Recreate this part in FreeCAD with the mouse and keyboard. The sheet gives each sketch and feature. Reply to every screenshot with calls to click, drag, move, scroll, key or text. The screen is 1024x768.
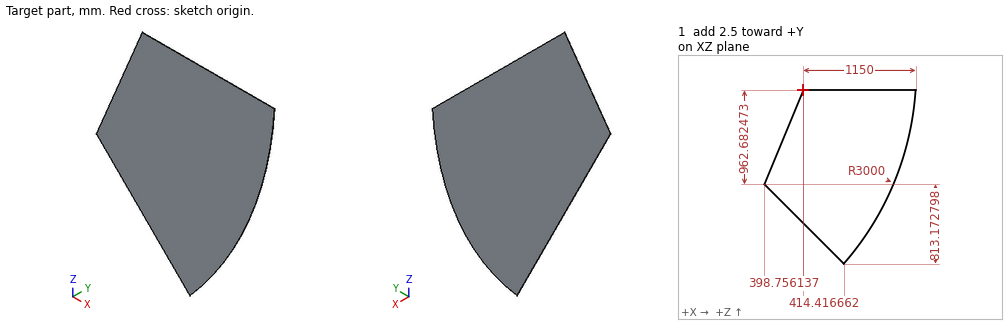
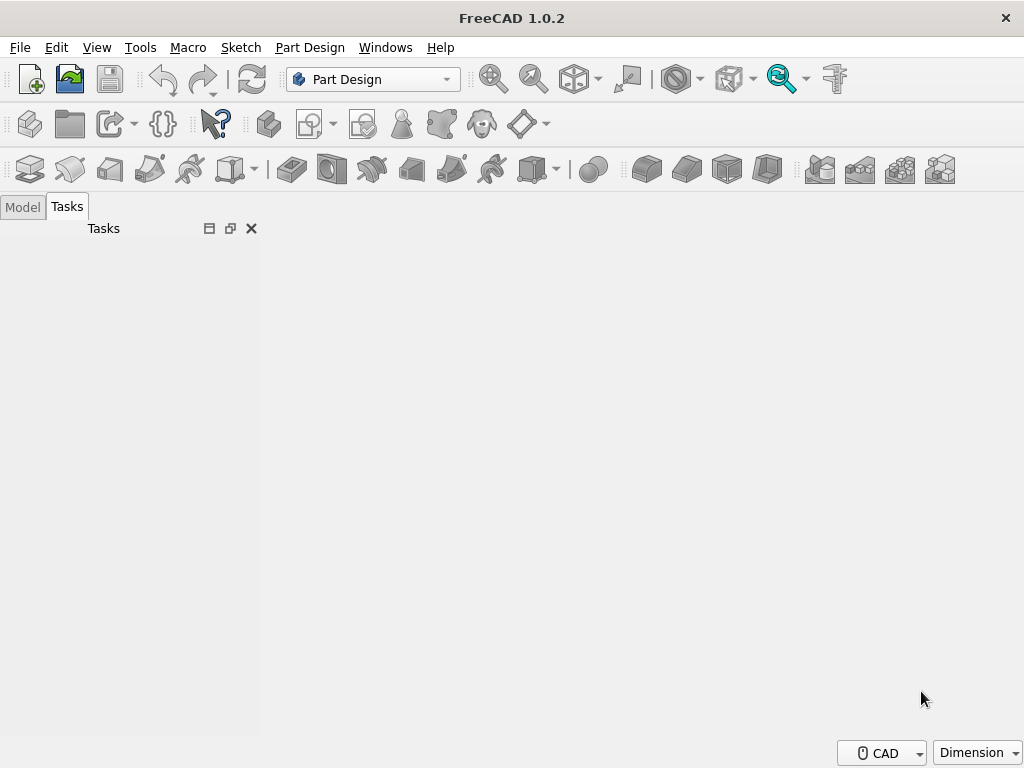
key(ctrl+n)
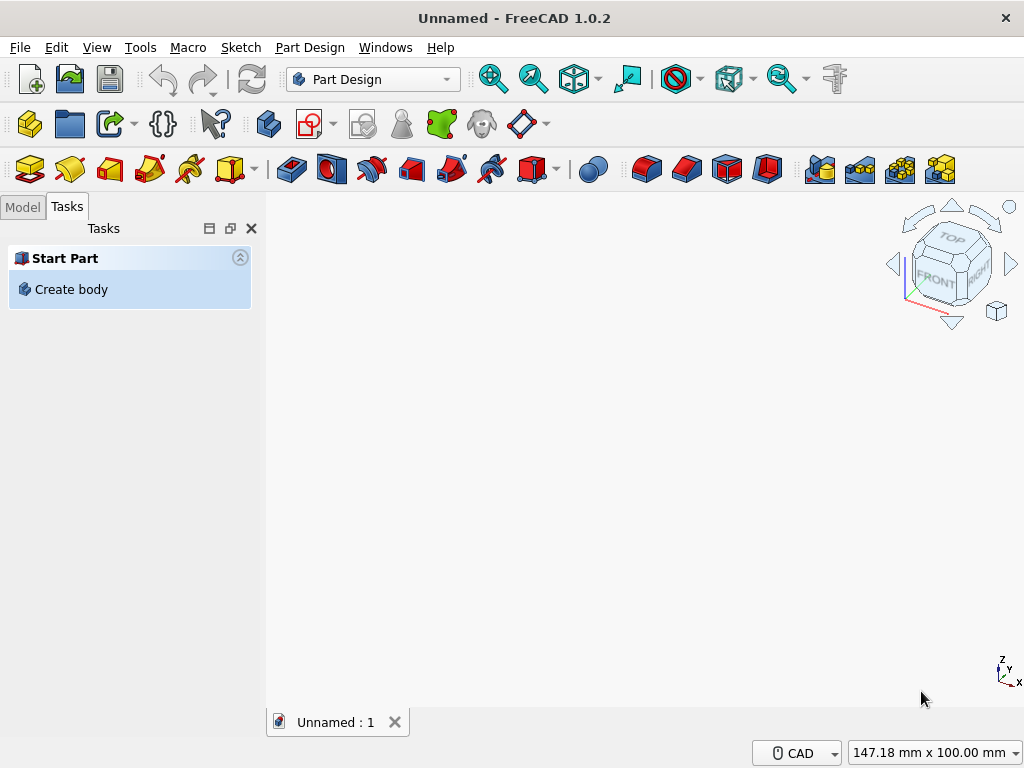
click(310, 124)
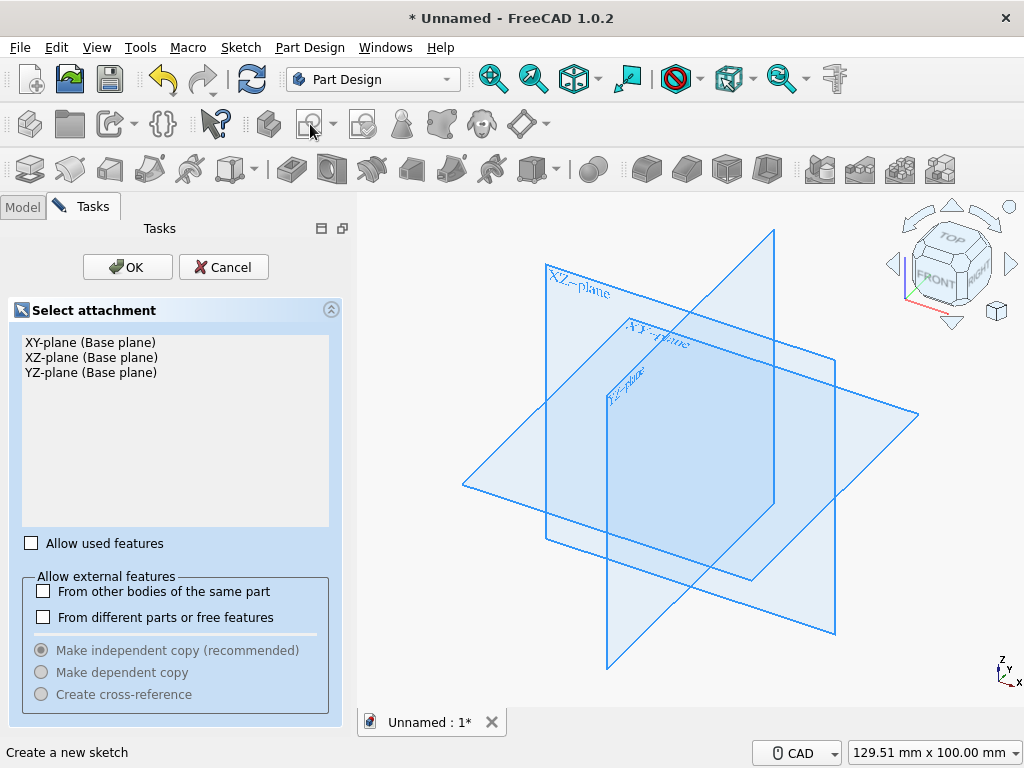
click(82, 358)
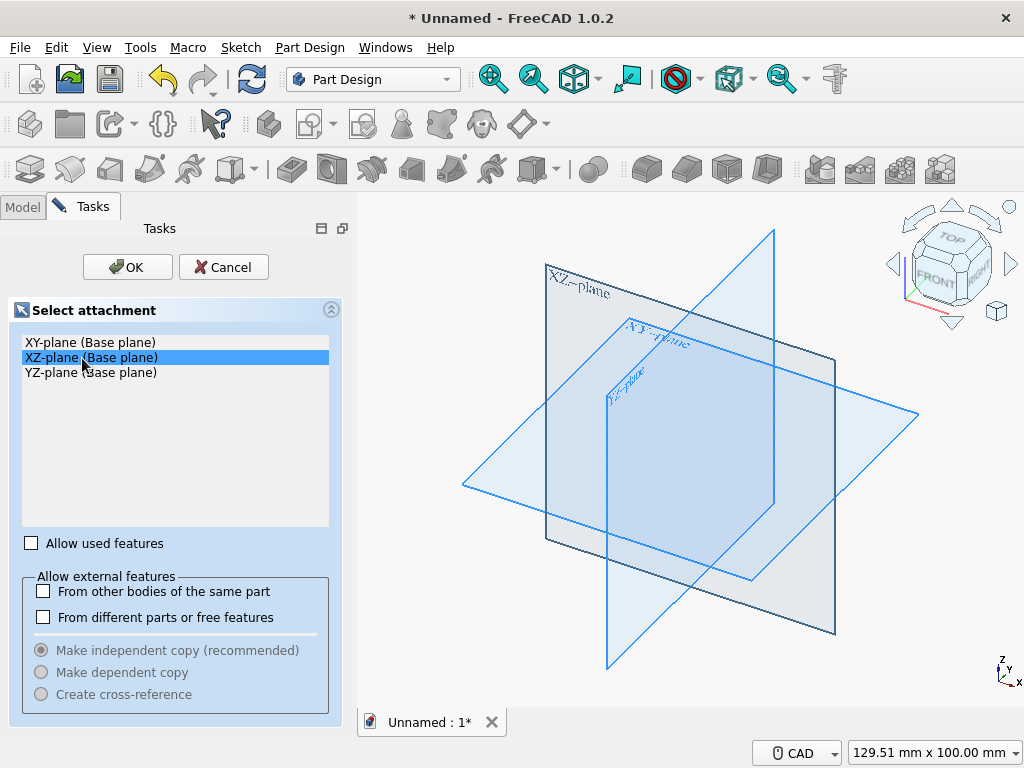
click(128, 267)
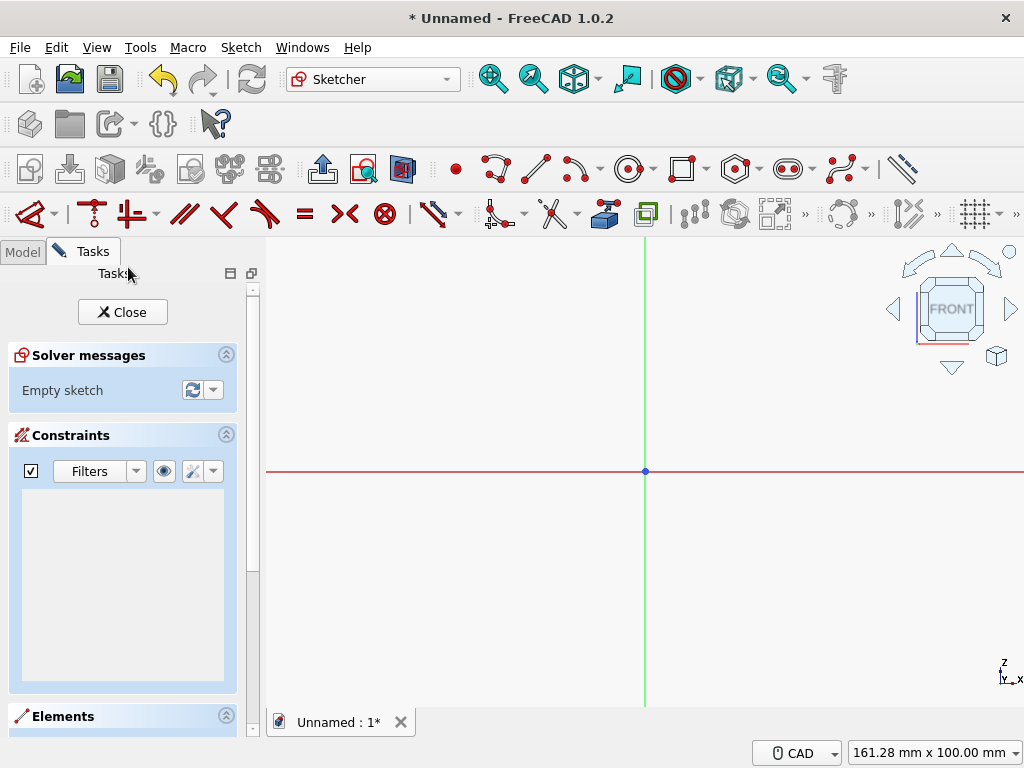
scroll(499, 295, down, 16)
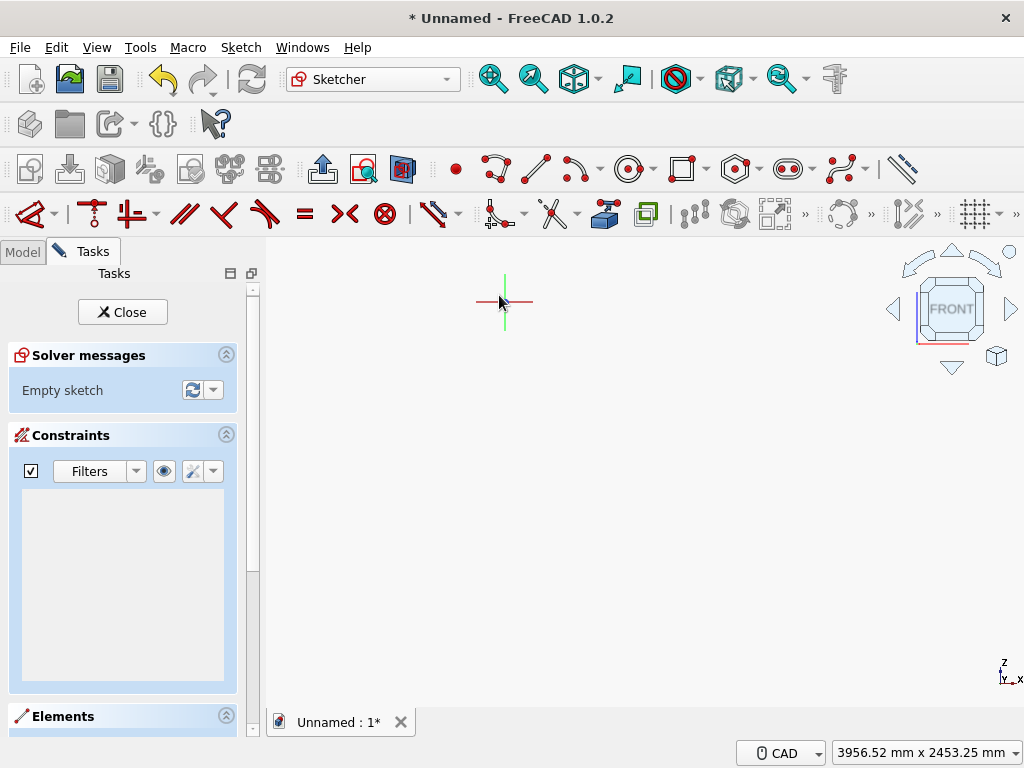
key(g)
key(m)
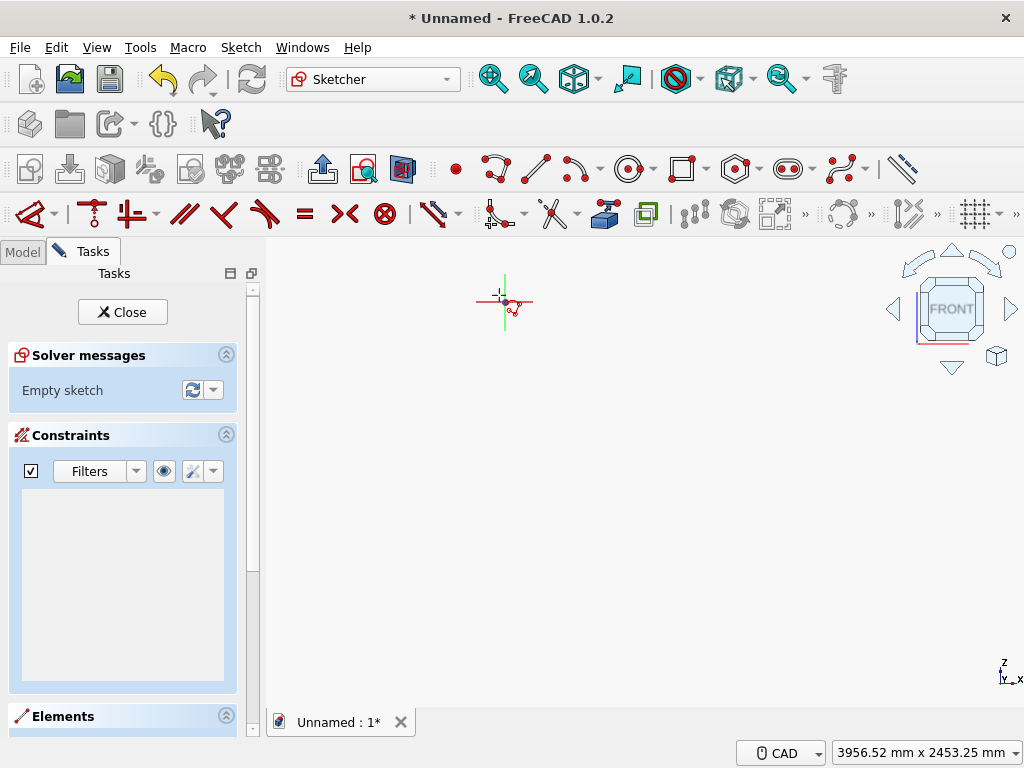
click(585, 643)
click(429, 487)
click(505, 302)
click(726, 311)
right_click(726, 311)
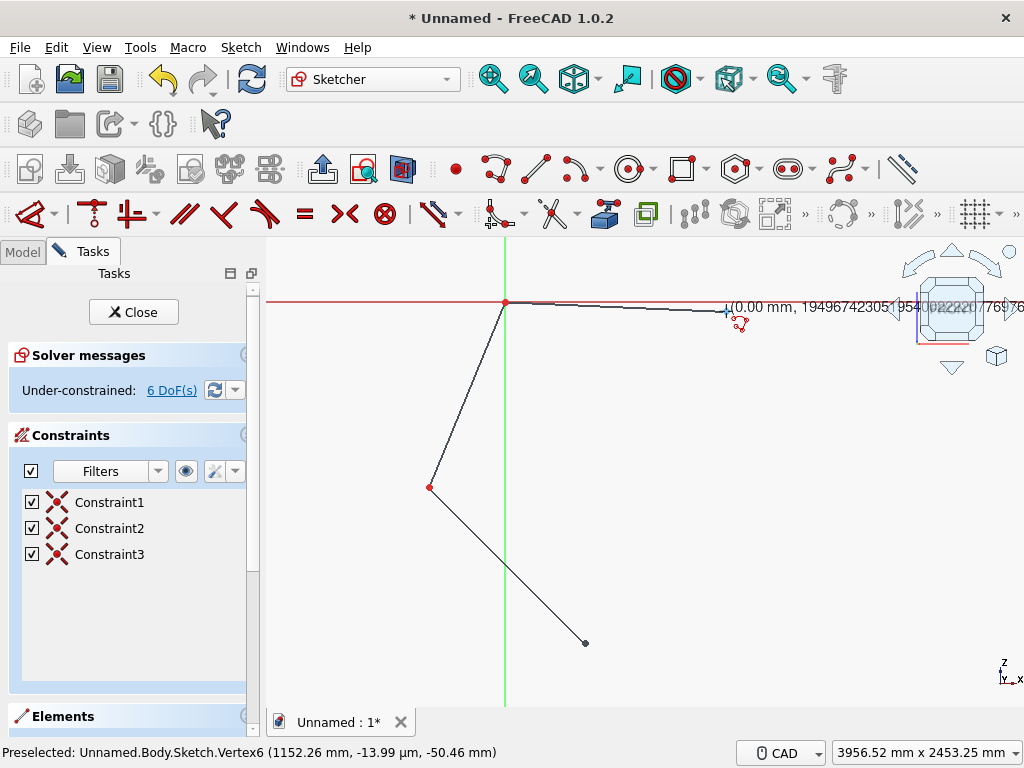
click(602, 170)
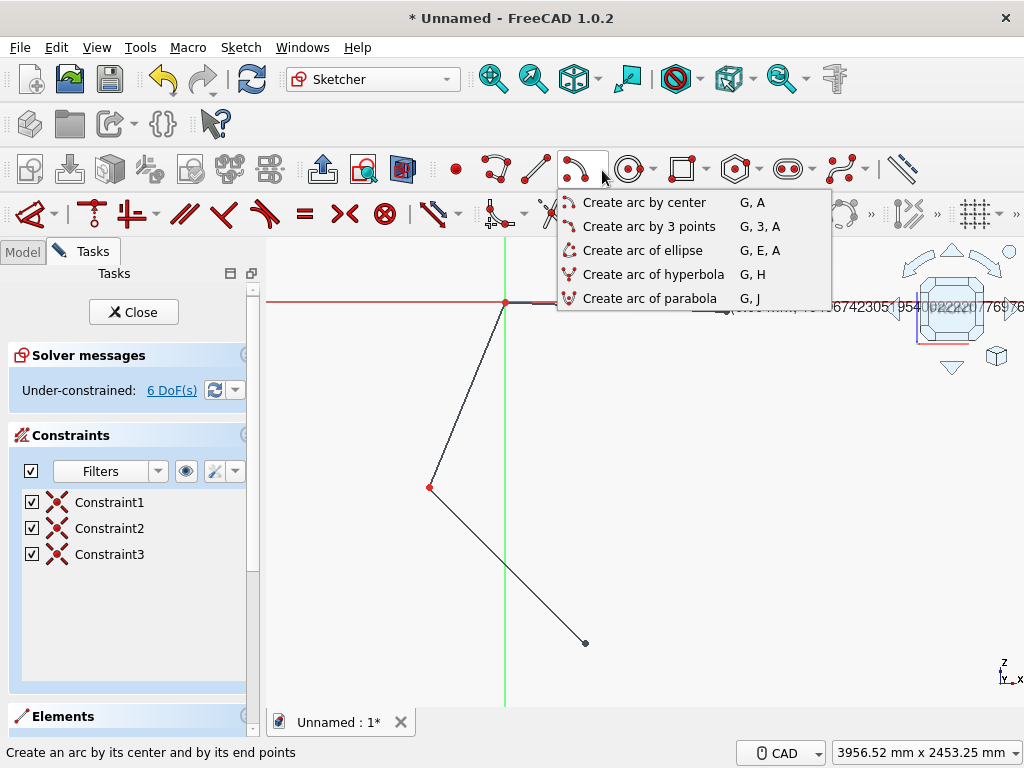
click(694, 226)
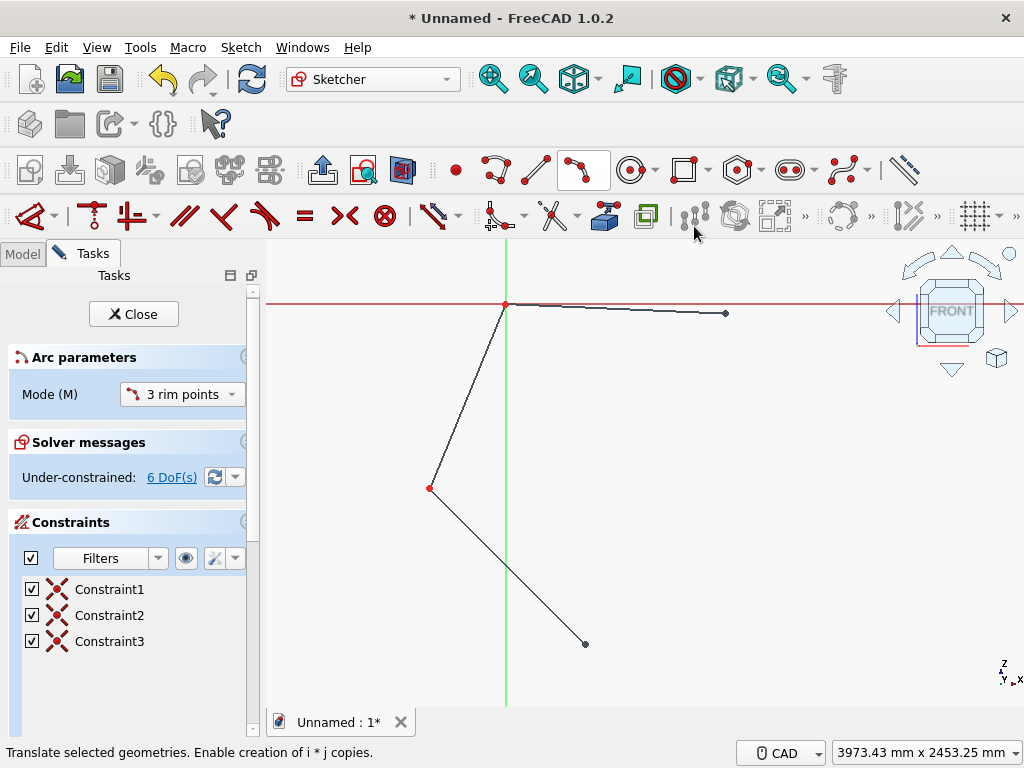
click(726, 314)
click(585, 644)
click(683, 485)
key(Escape)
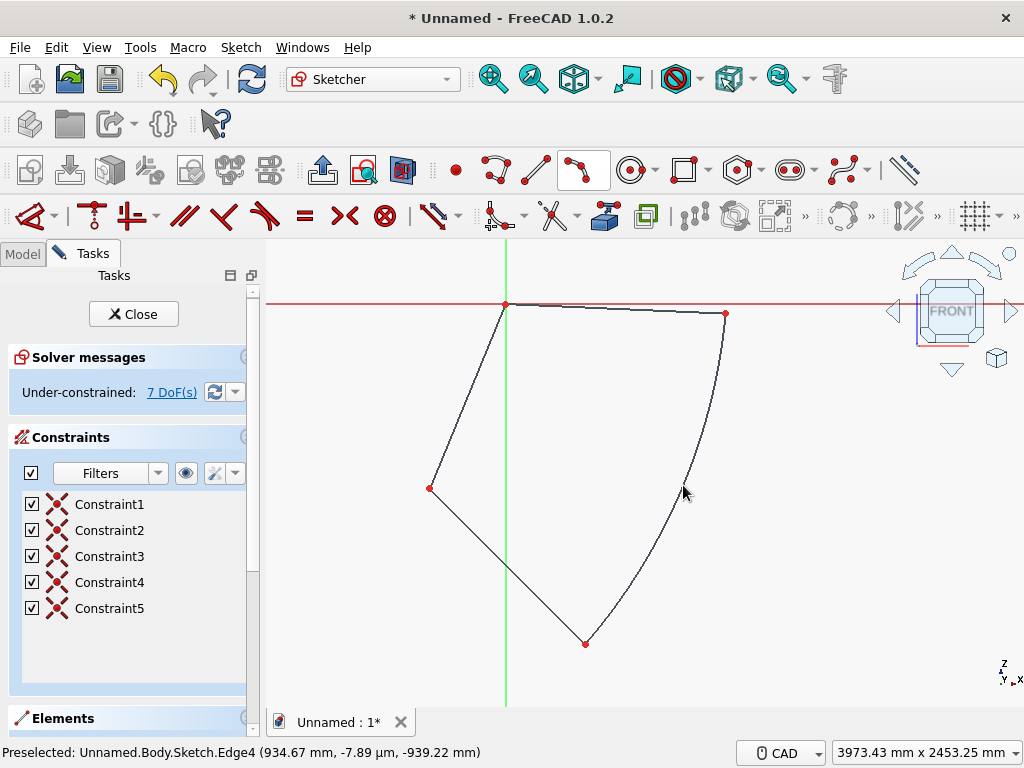
click(572, 307)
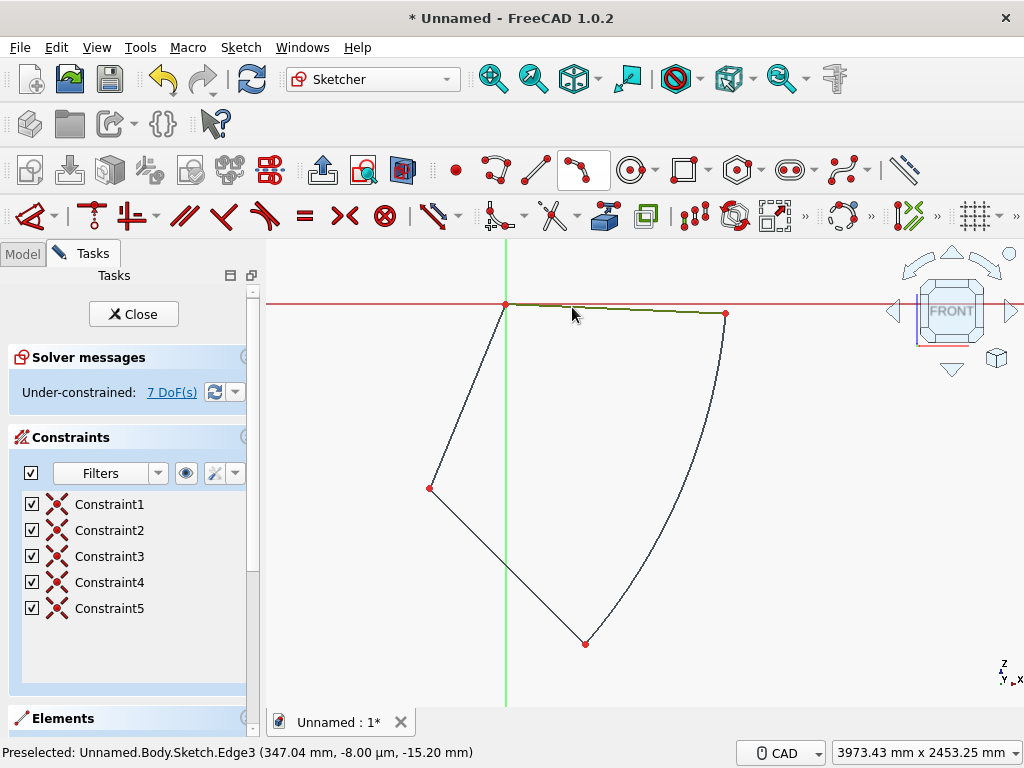
key(h)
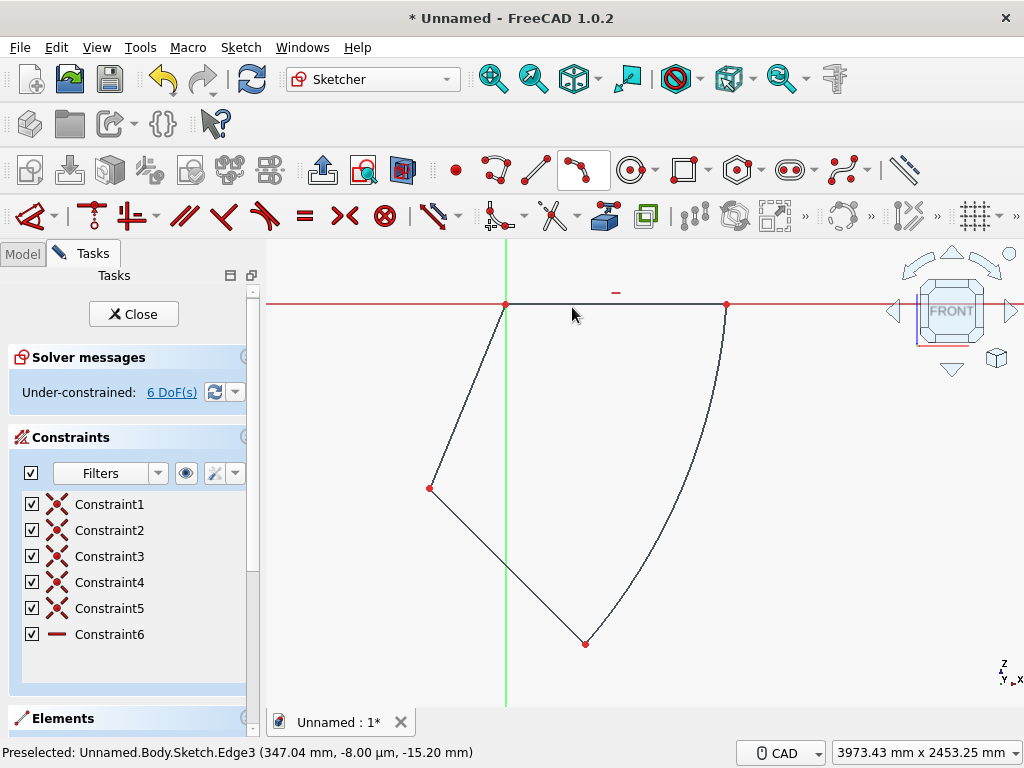
click(650, 553)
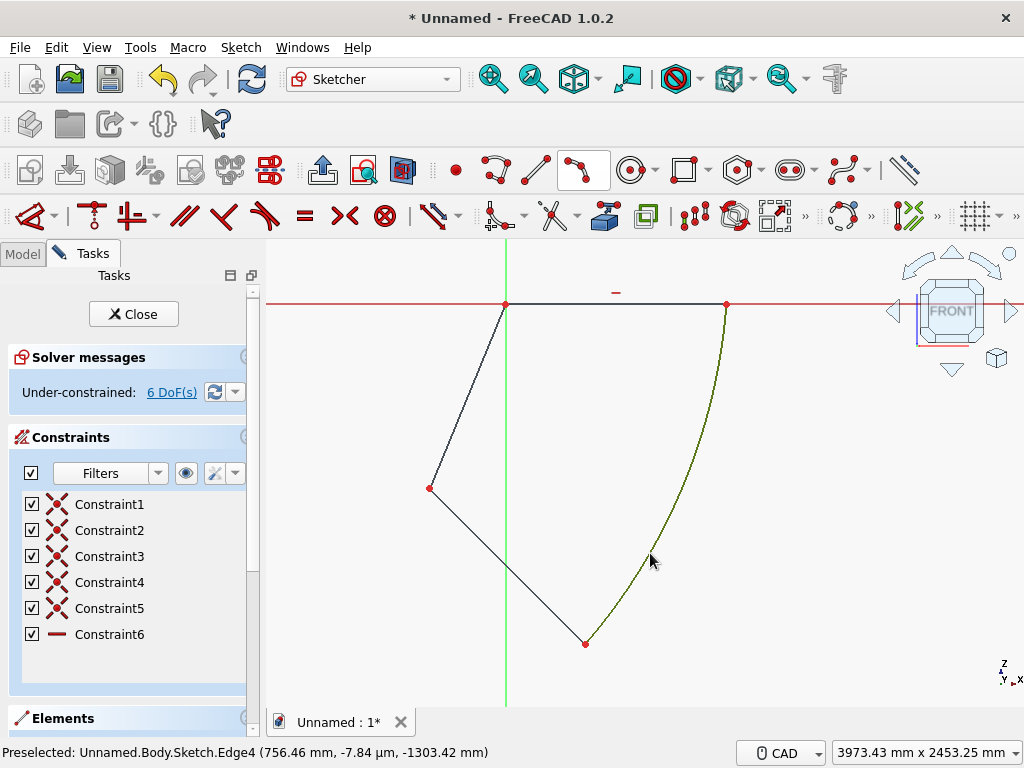
key(k)
key(r)